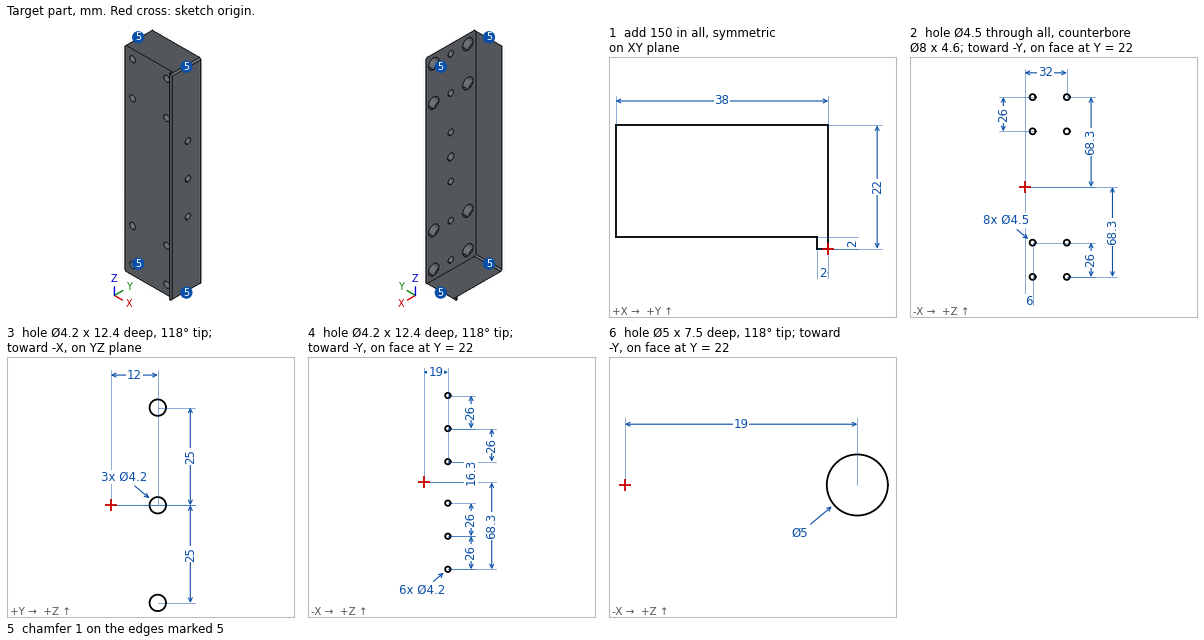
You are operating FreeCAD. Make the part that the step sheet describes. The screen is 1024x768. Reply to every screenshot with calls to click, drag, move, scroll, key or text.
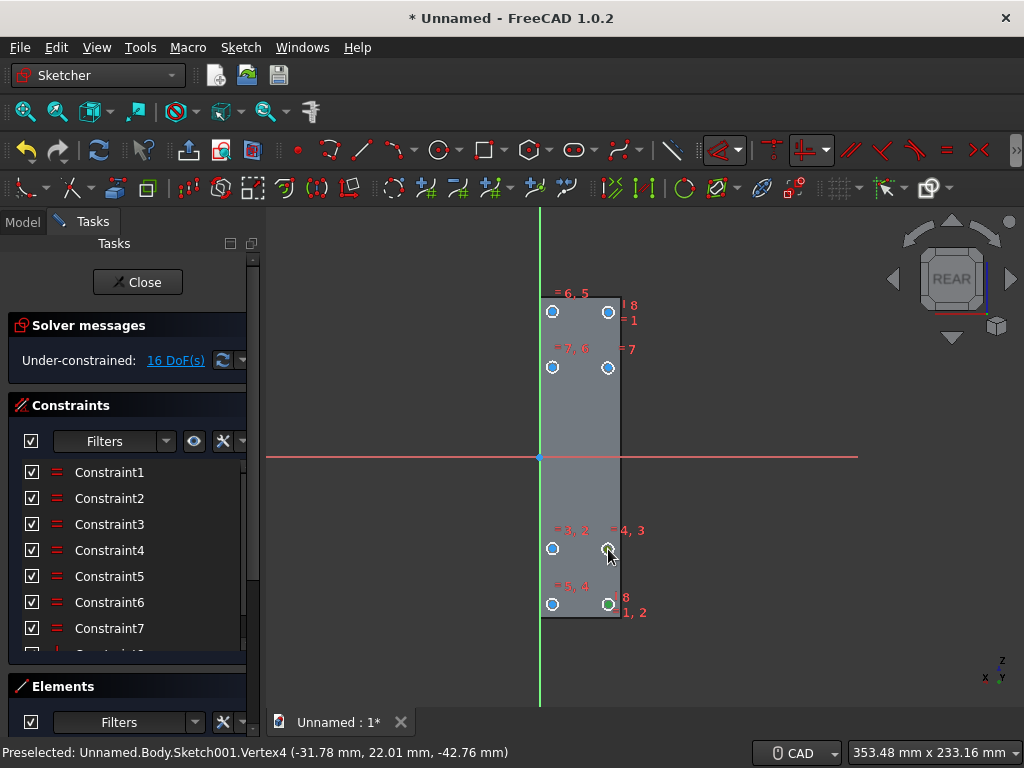
key(v)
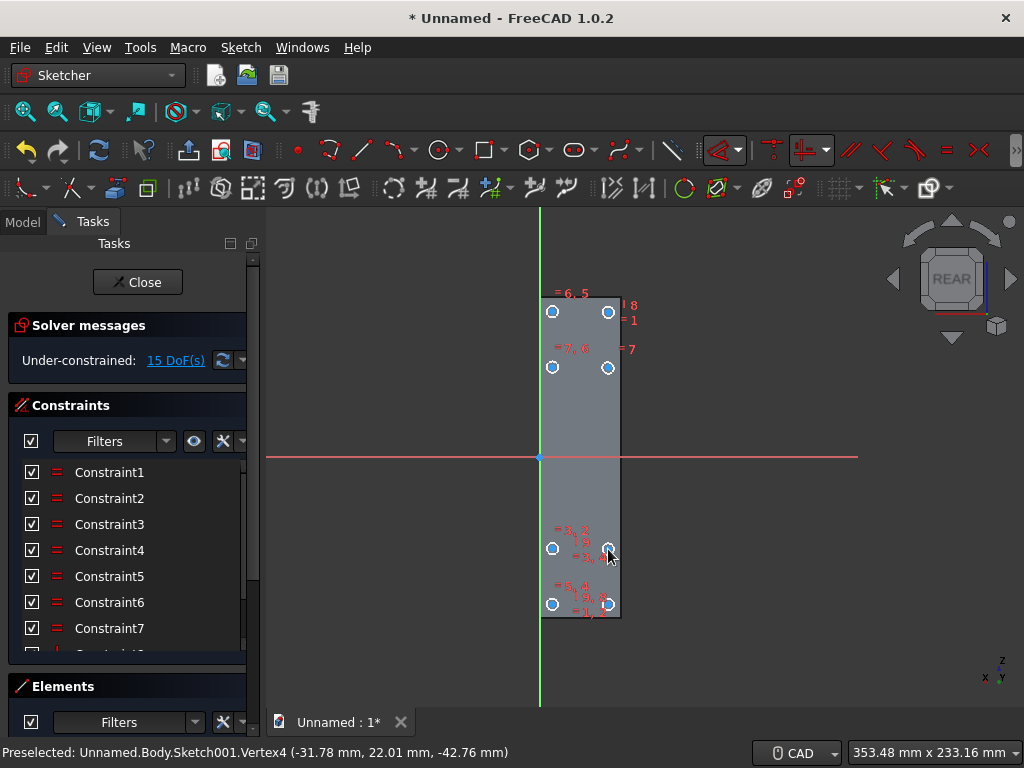
click(553, 549)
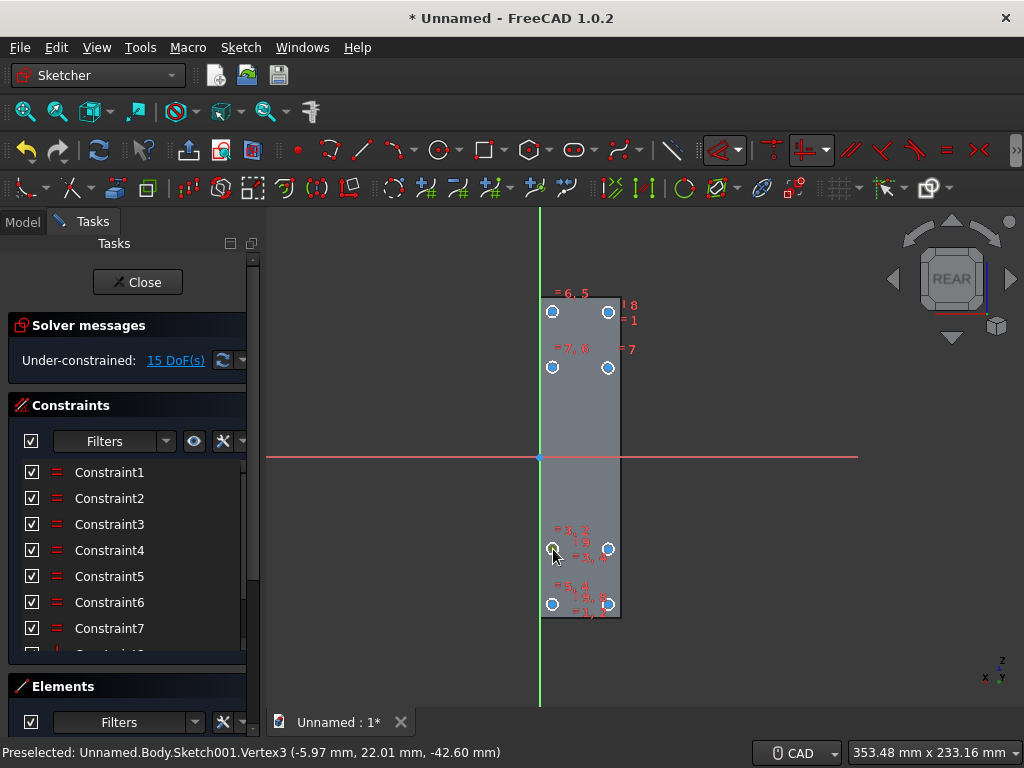
click(608, 549)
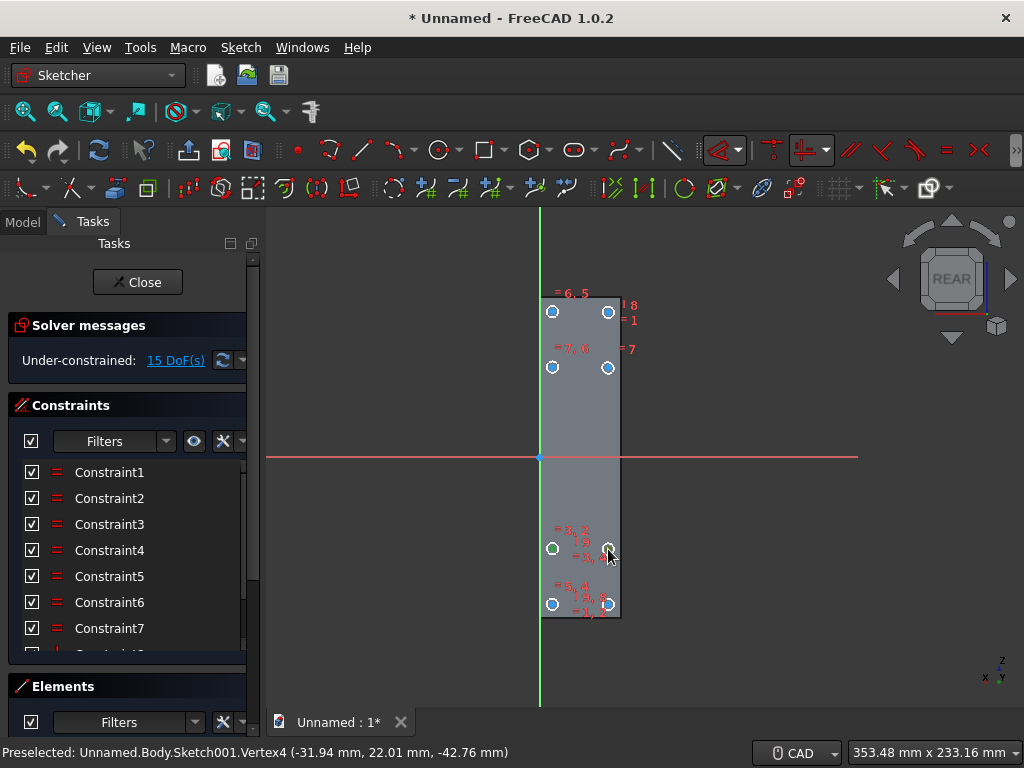
click(828, 150)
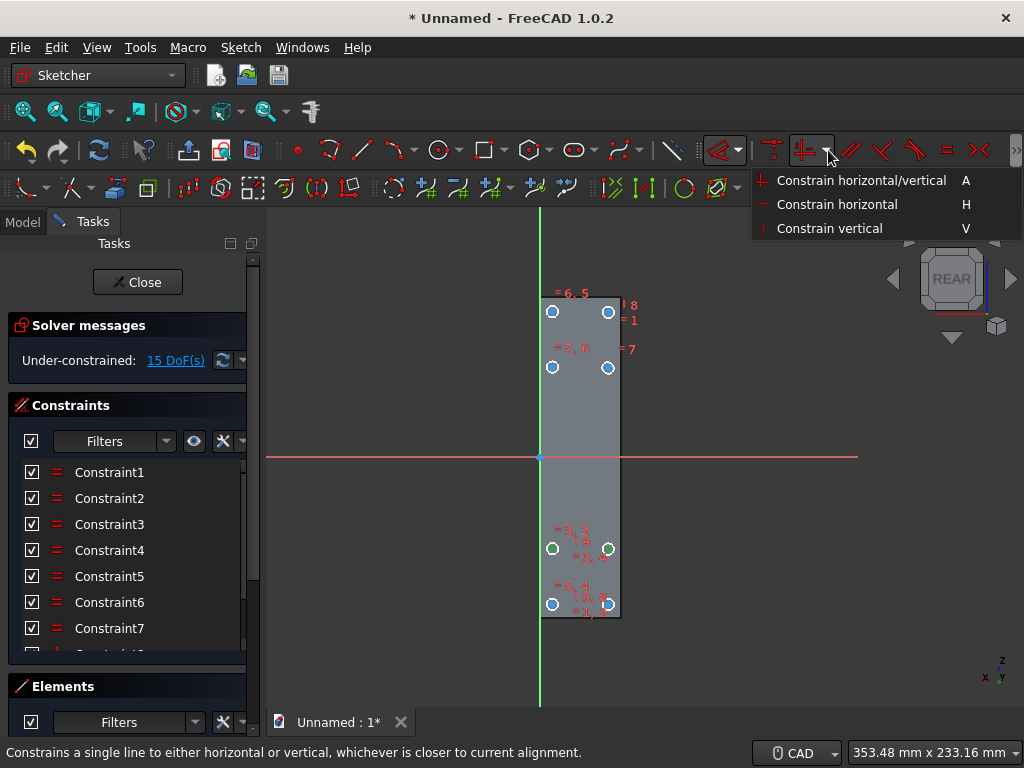
click(887, 204)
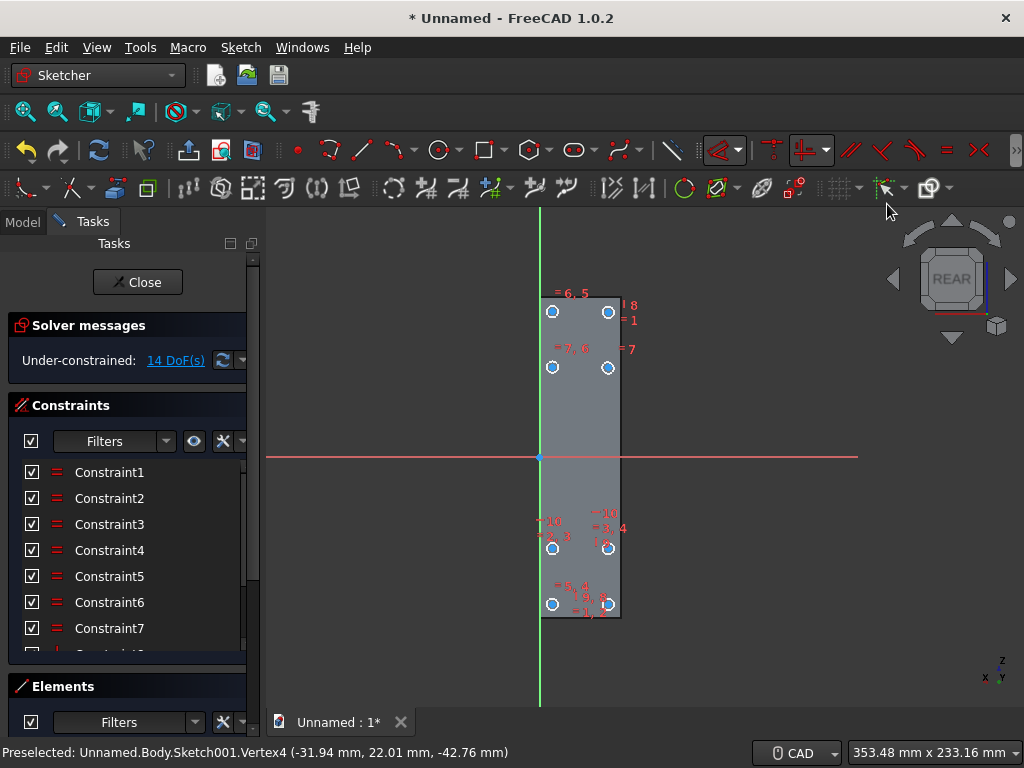
click(553, 549)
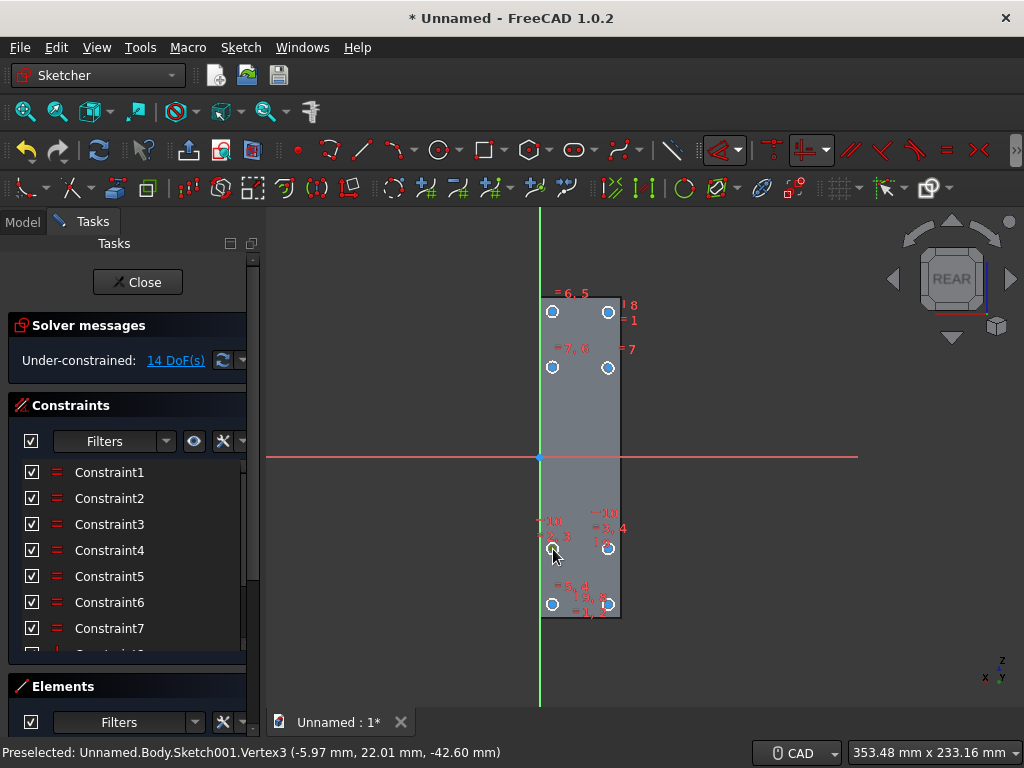
click(552, 604)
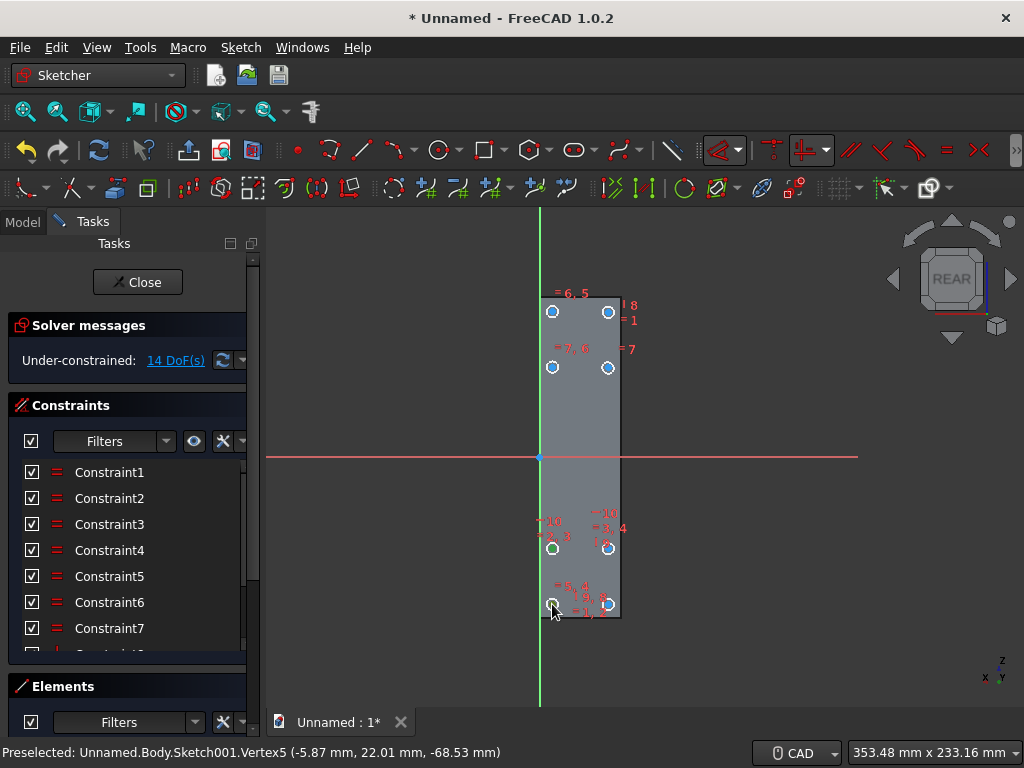
key(v)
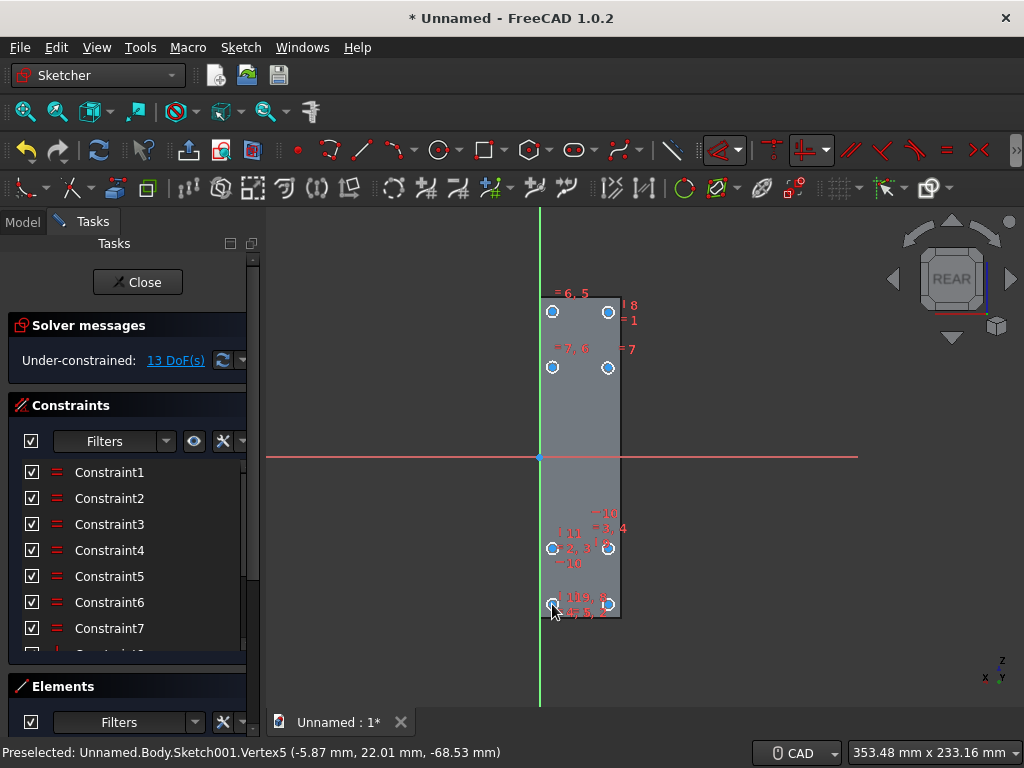
click(608, 604)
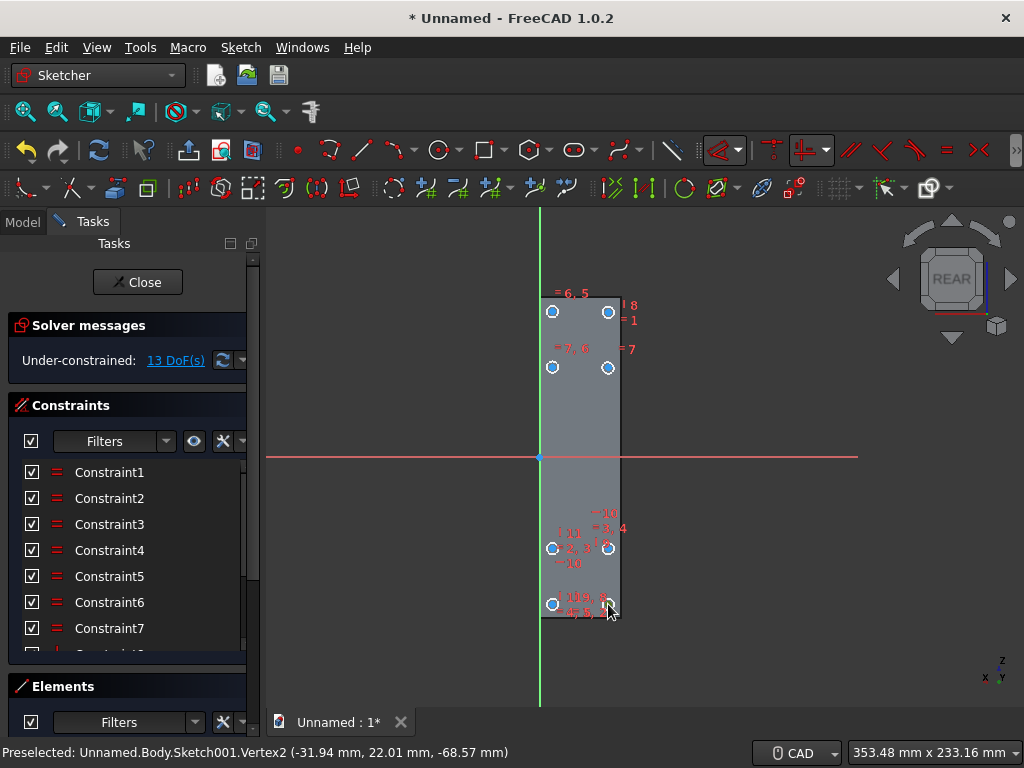
click(553, 604)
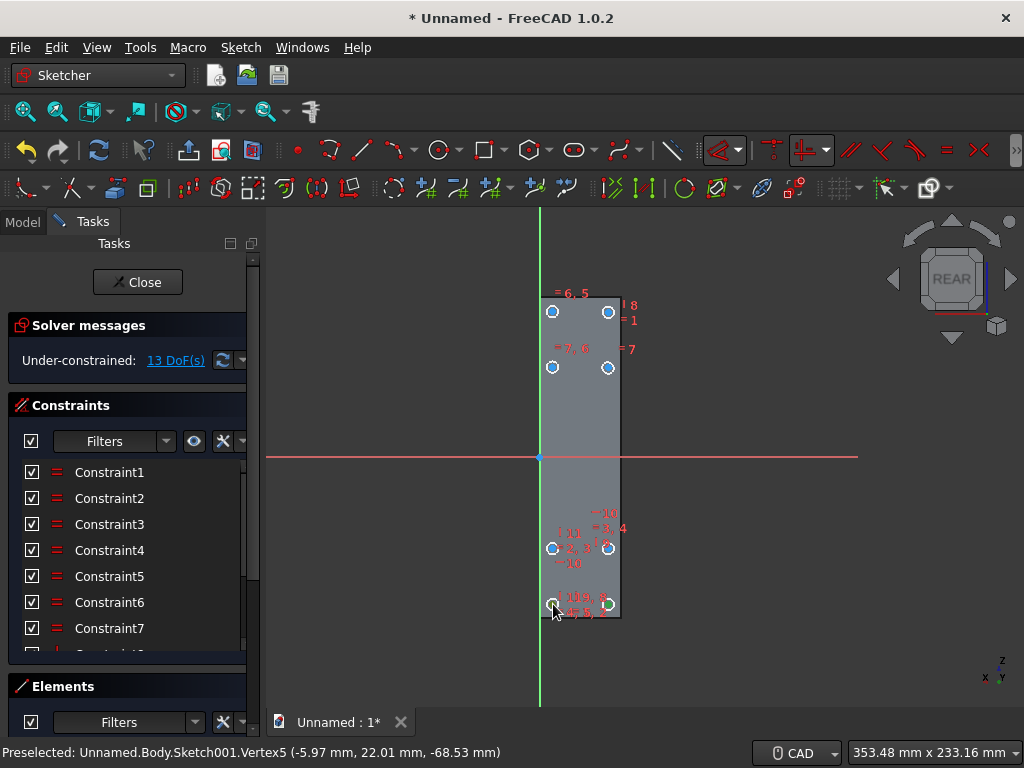
key(h)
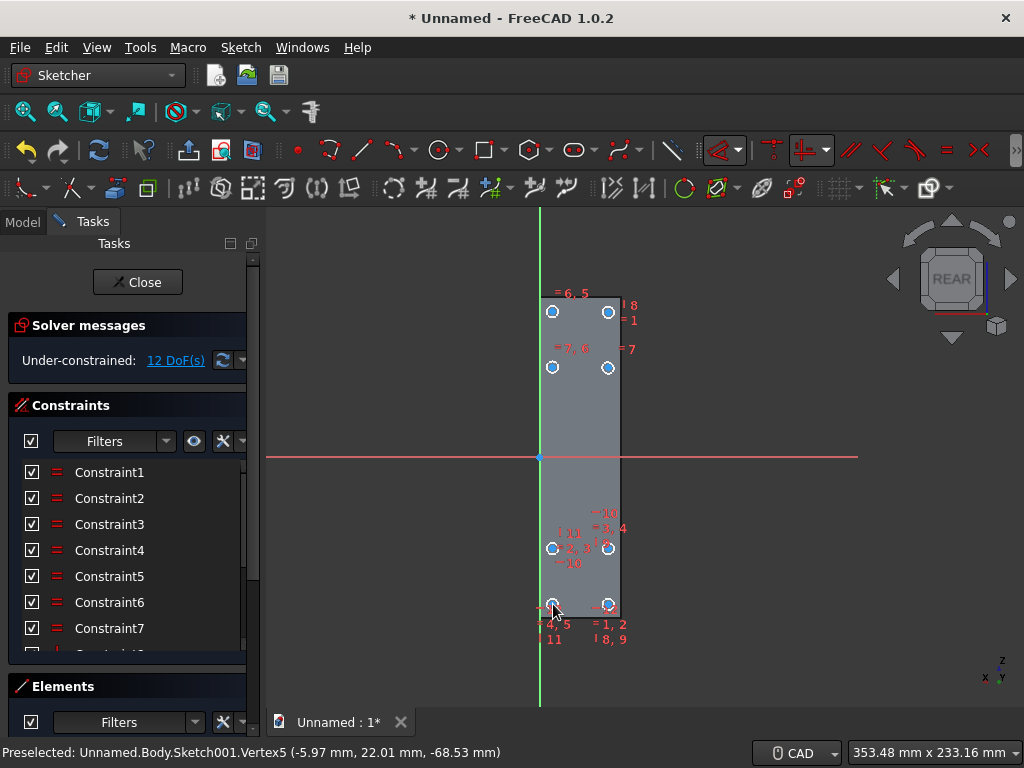
click(553, 549)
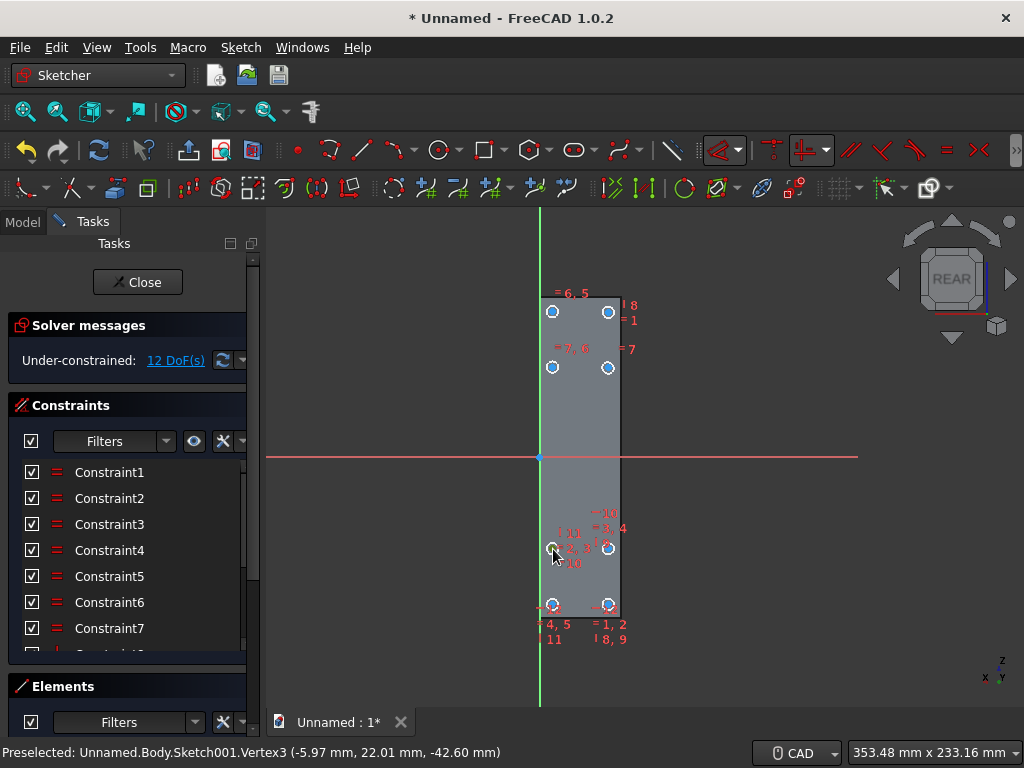
click(552, 312)